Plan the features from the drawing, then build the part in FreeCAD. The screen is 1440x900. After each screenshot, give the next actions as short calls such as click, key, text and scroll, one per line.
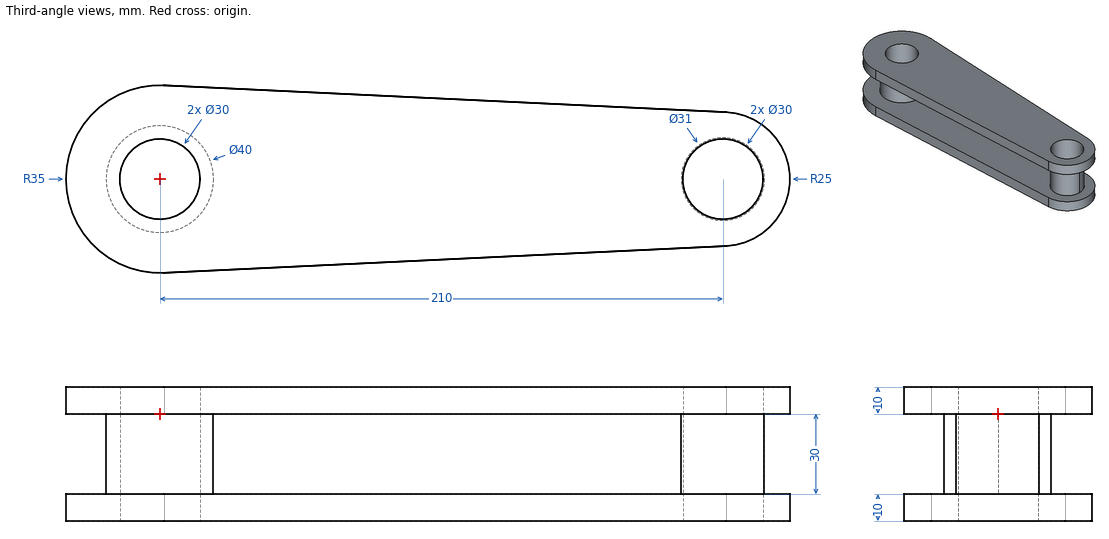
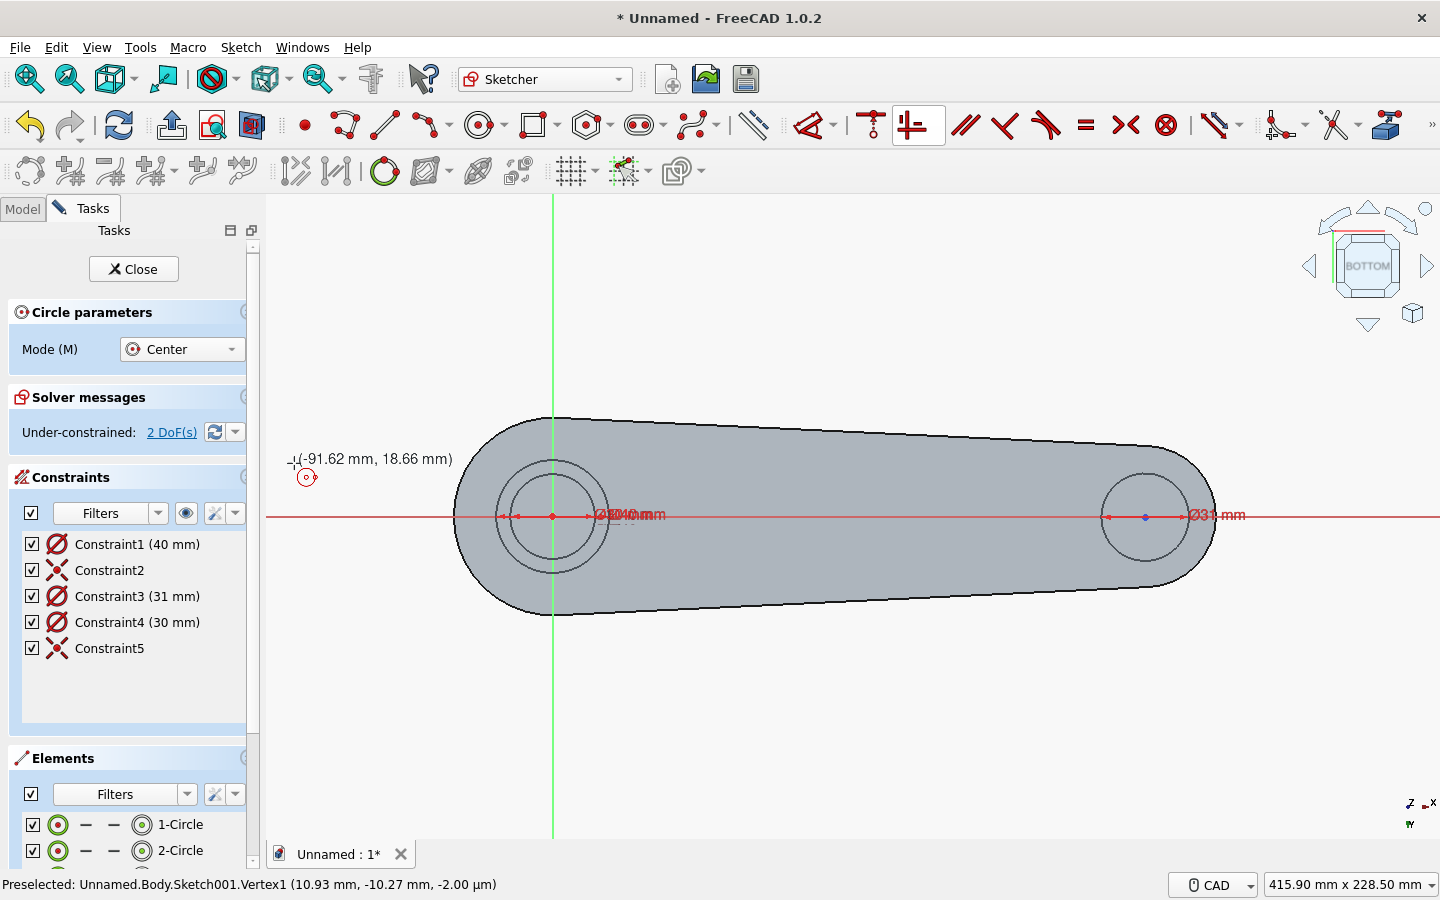
click(1145, 517)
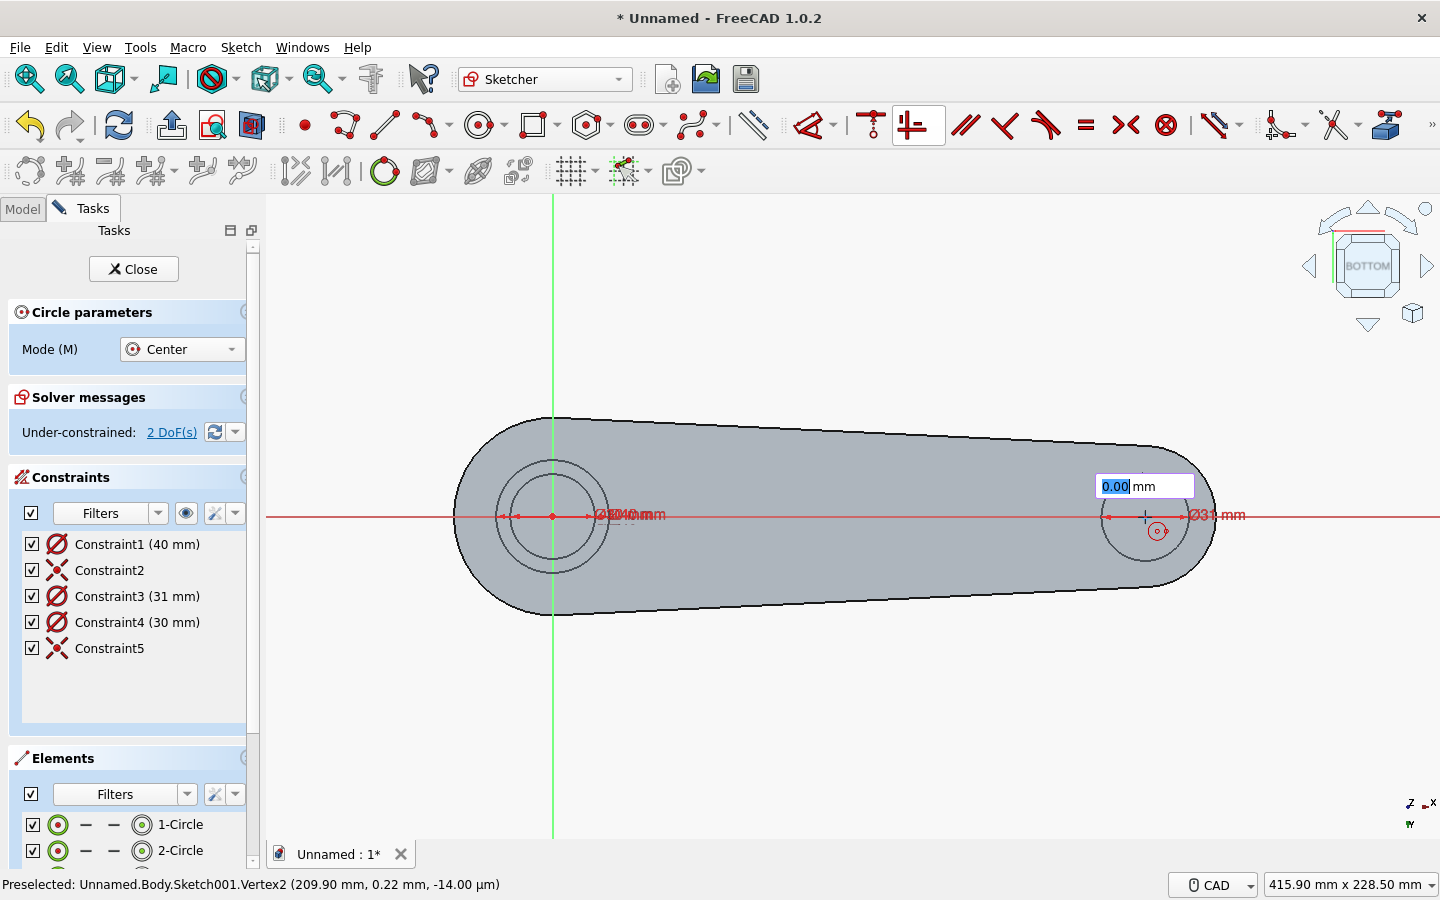
scroll(1175, 487, up, 13)
move(1170, 476)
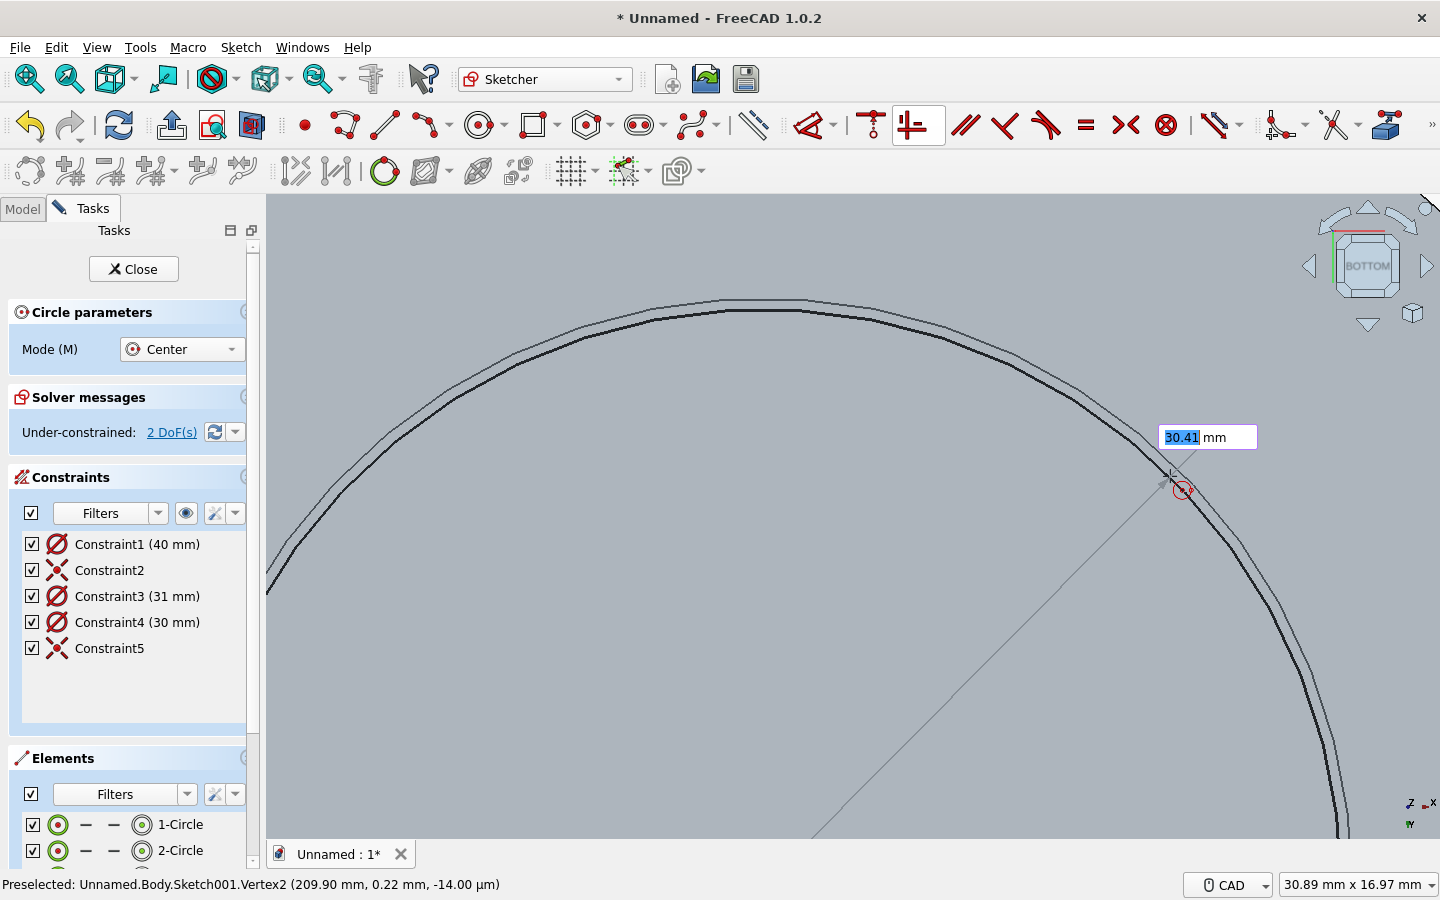
text(30)
key(Return)
key(Escape)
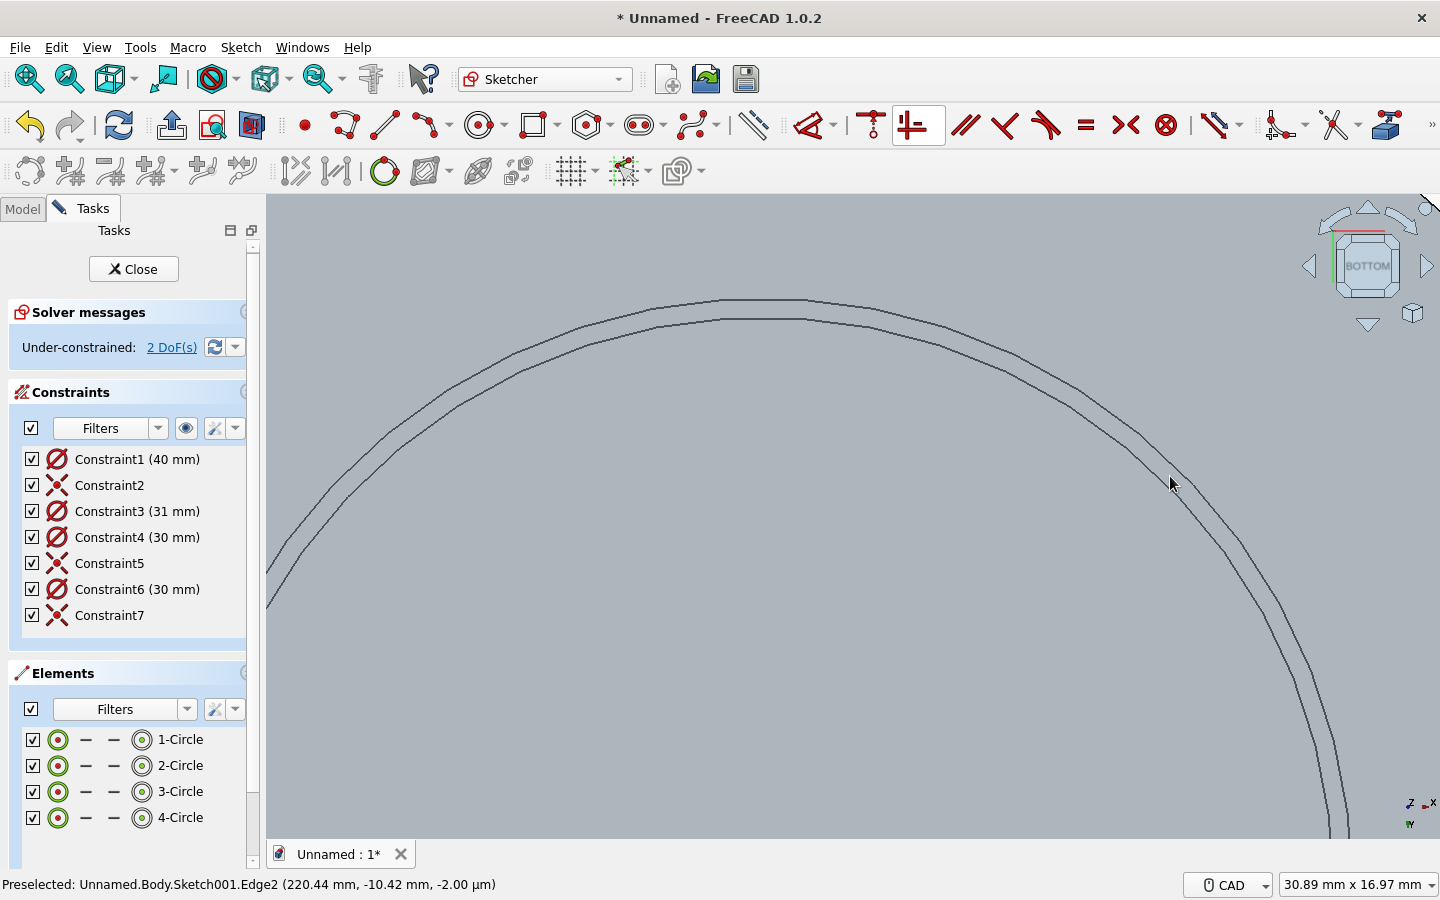
scroll(1113, 487, down, 13)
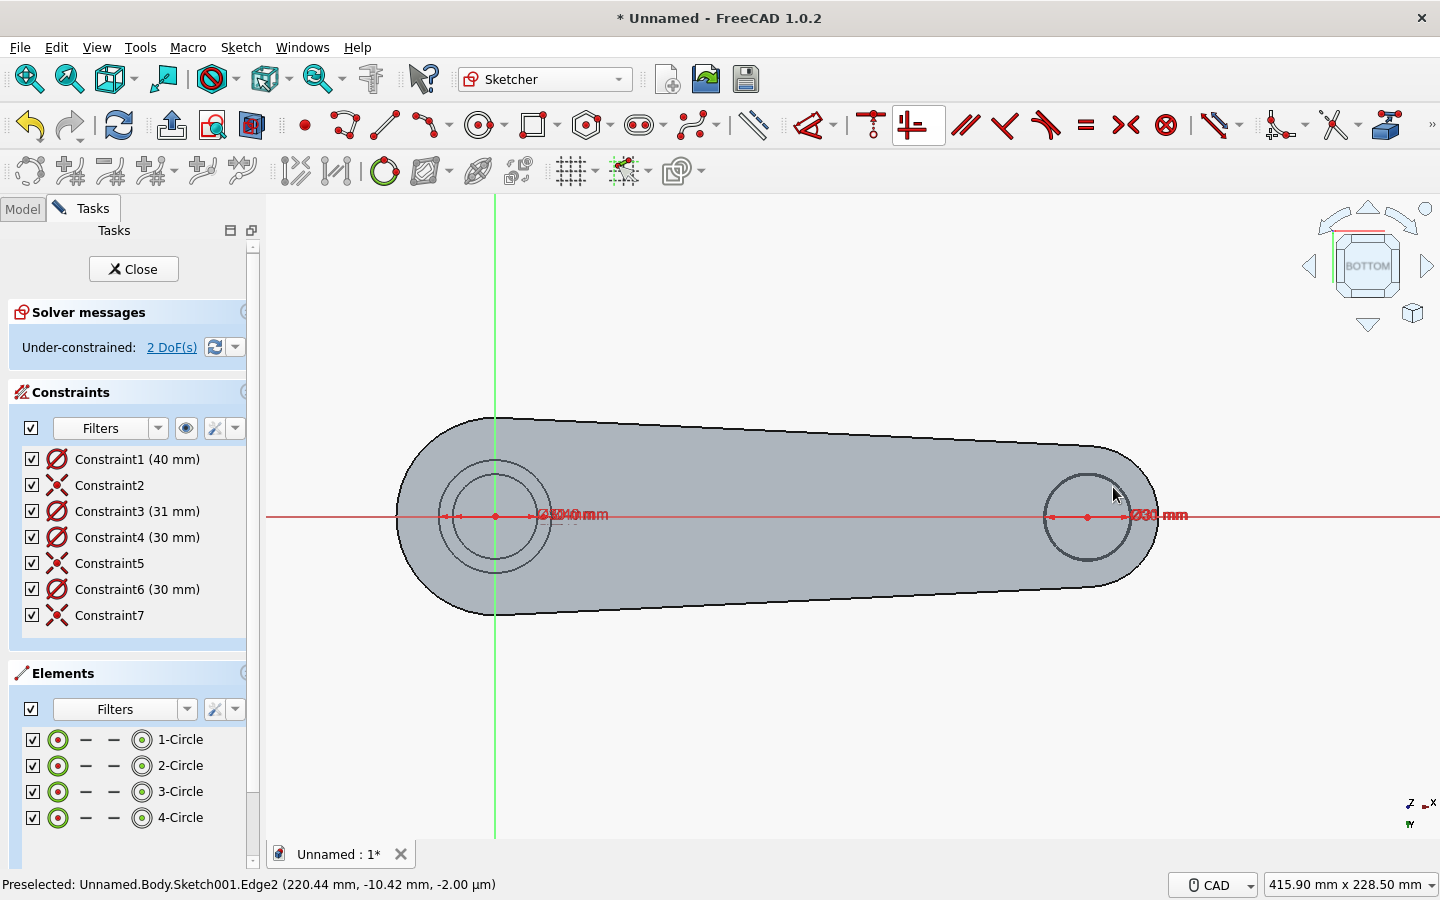
click(1088, 517)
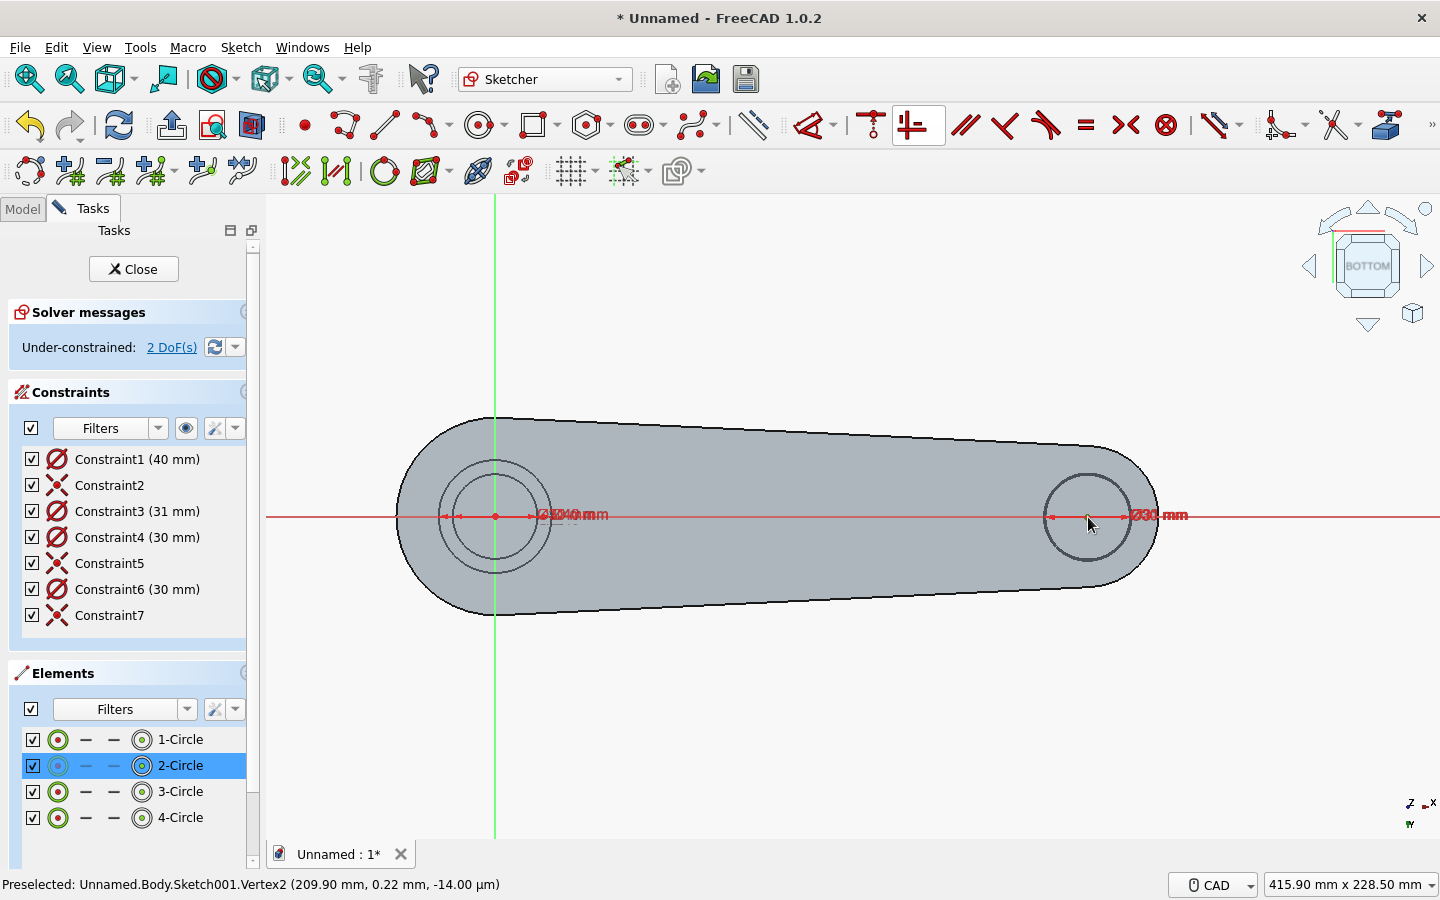
click(364, 517)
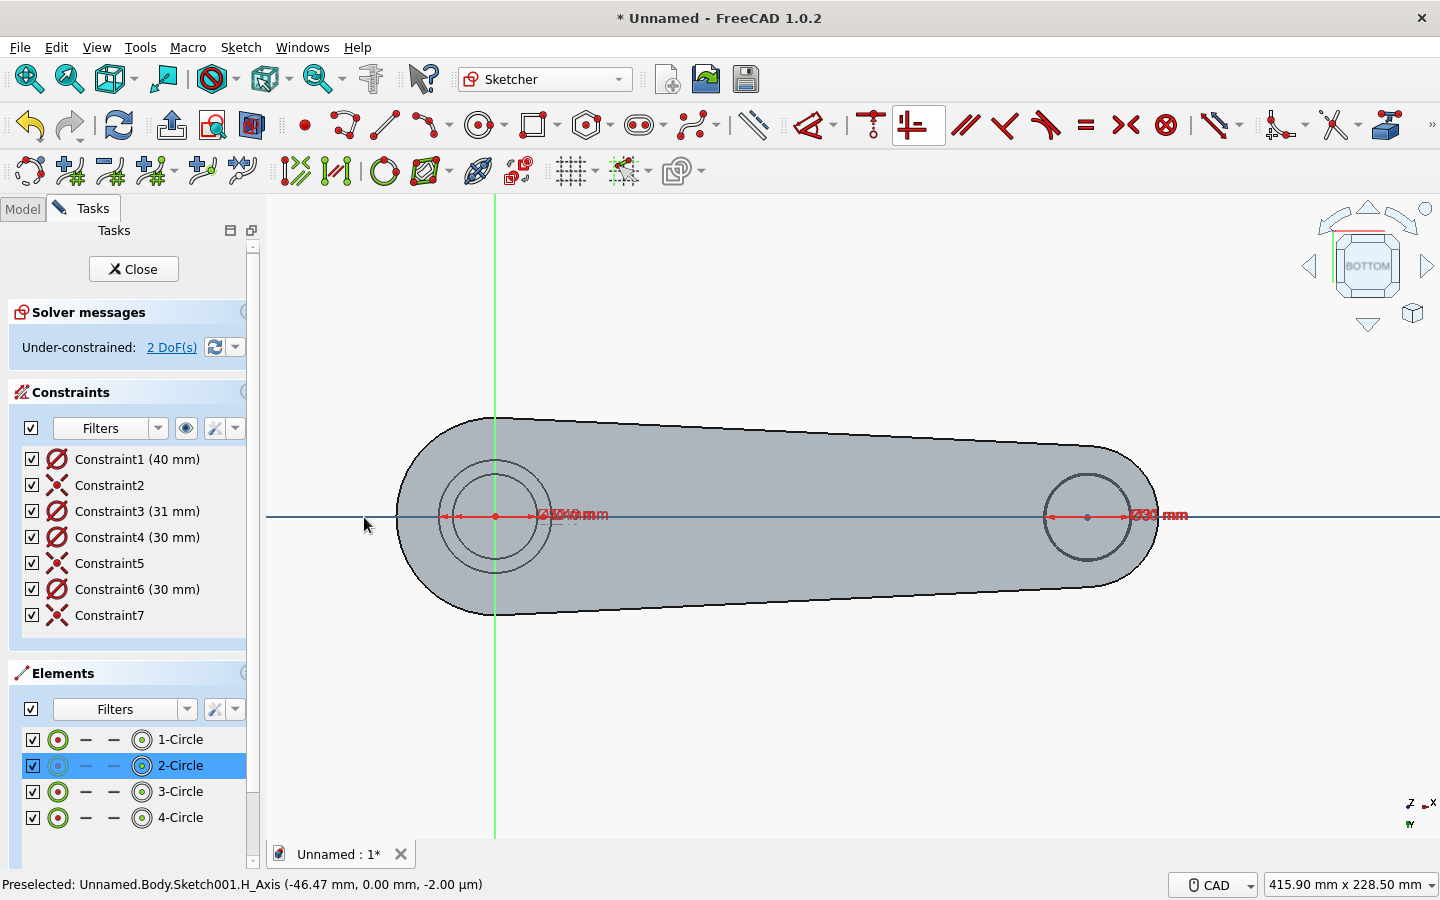
click(872, 126)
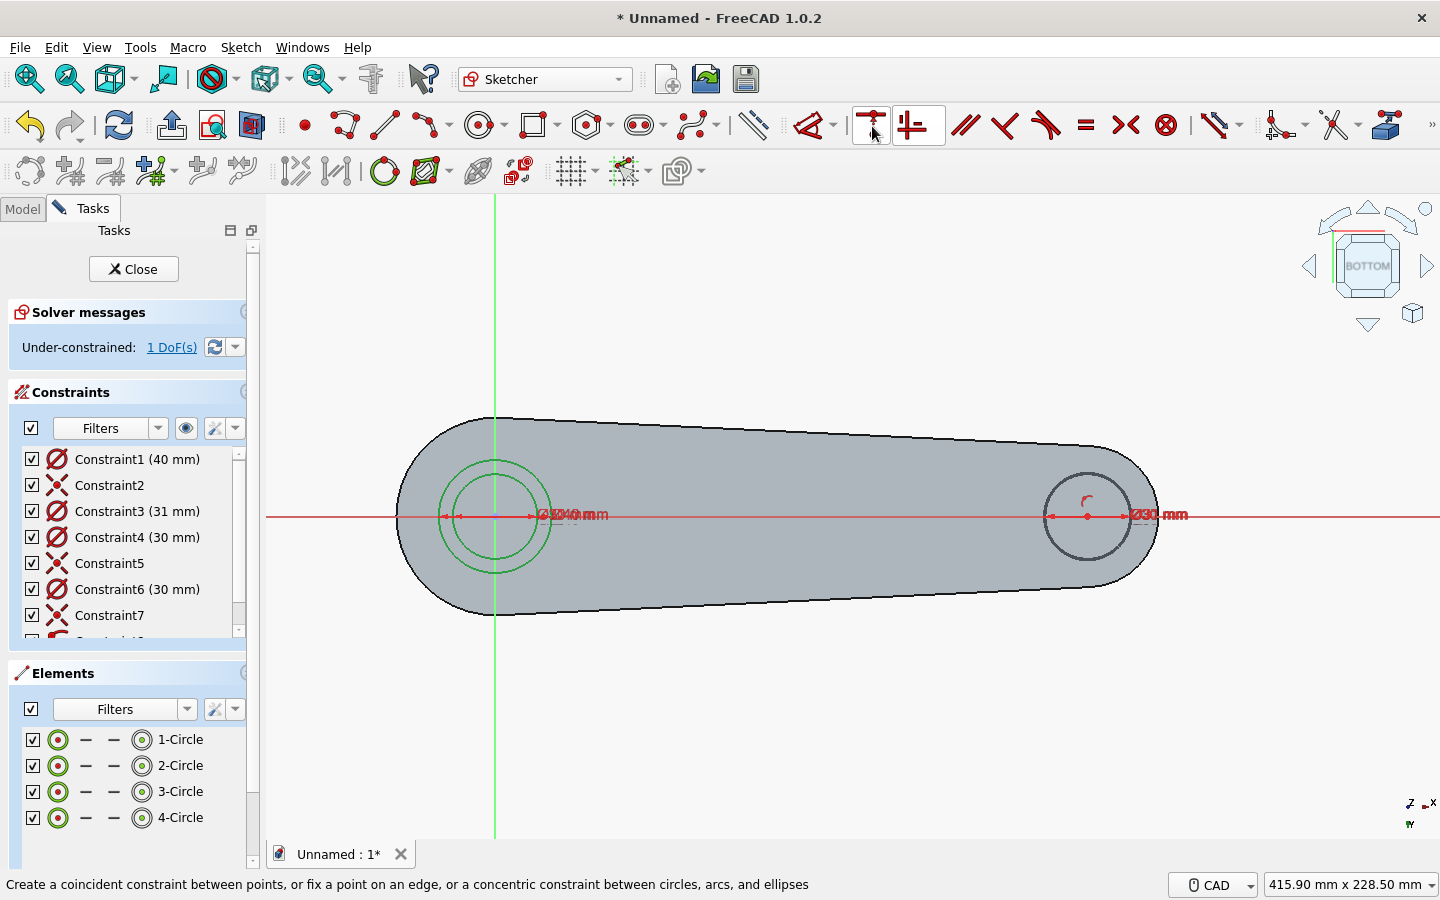
click(808, 126)